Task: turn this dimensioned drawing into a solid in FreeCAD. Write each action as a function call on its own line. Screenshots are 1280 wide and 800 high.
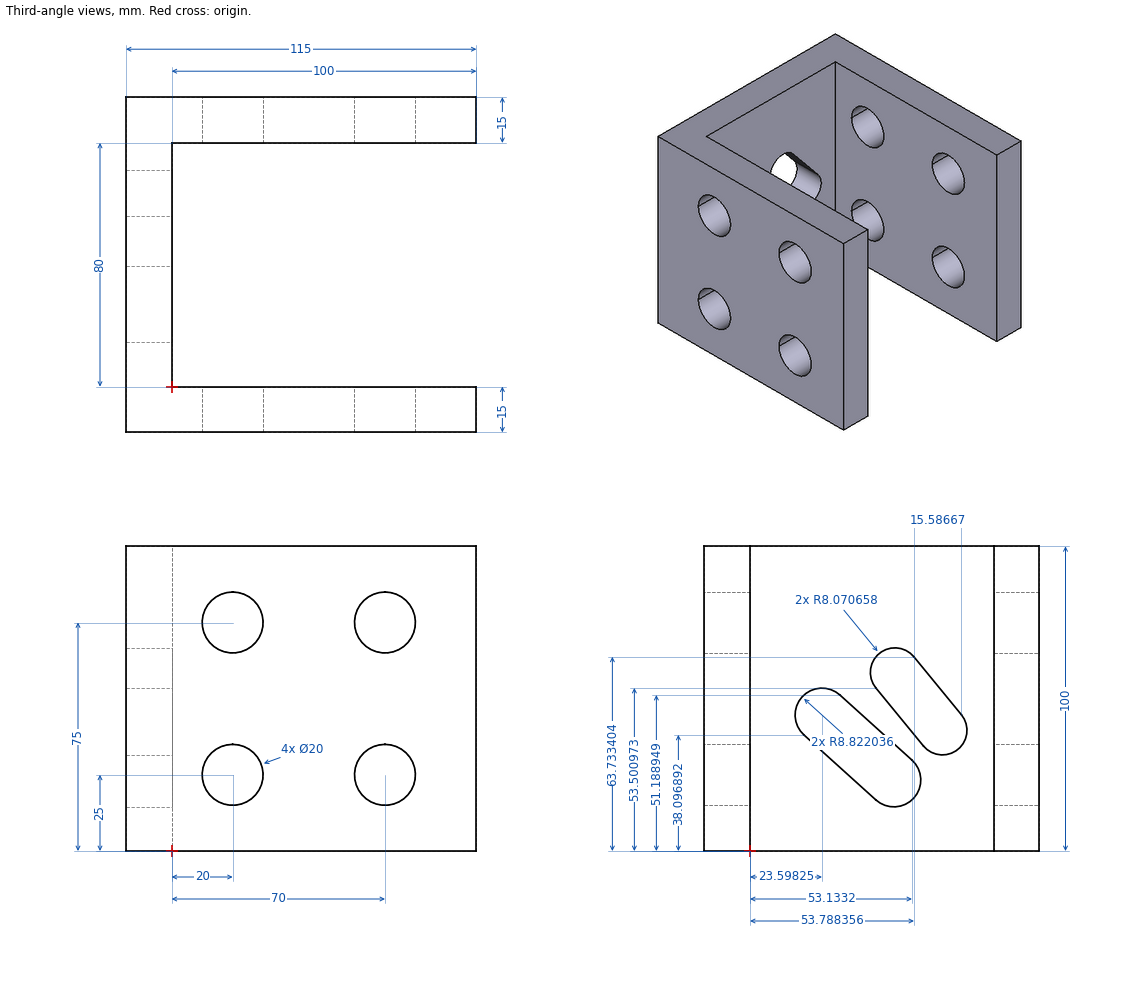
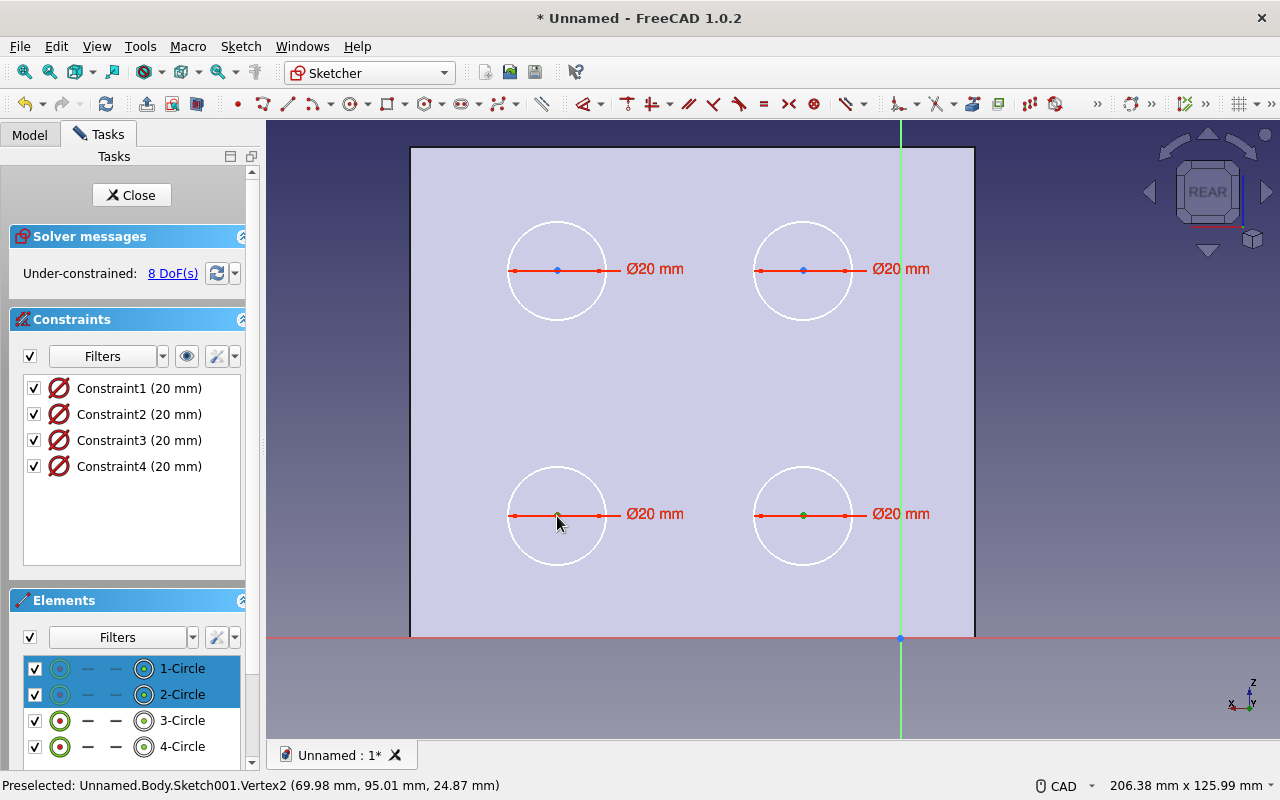
key(h)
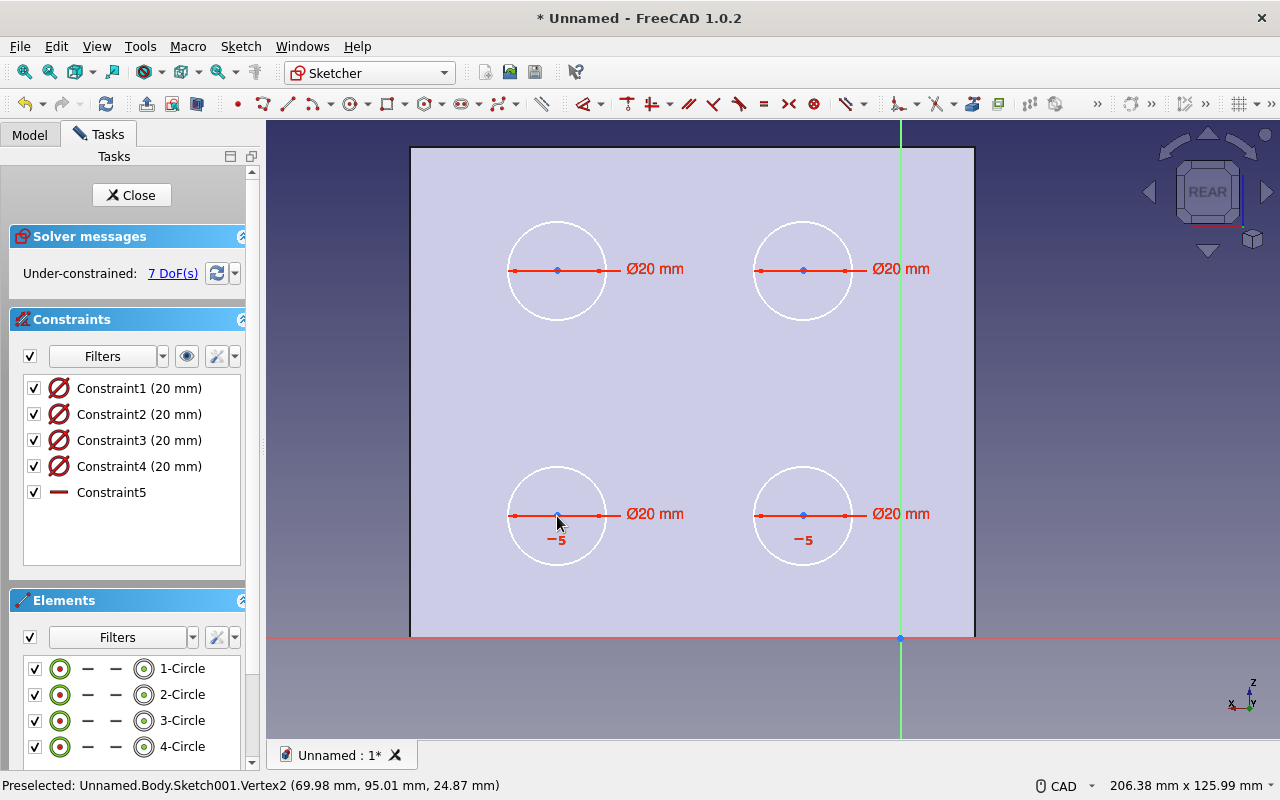
click(803, 516)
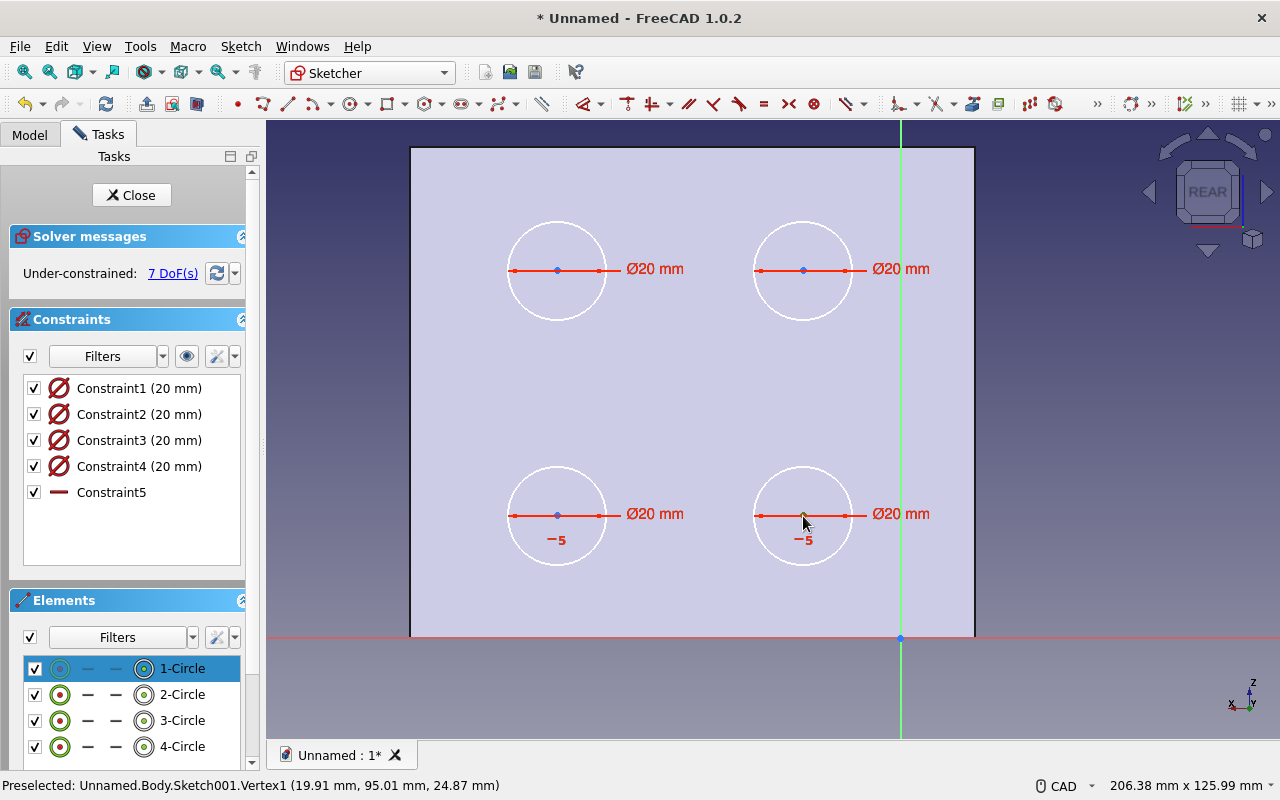
click(803, 271)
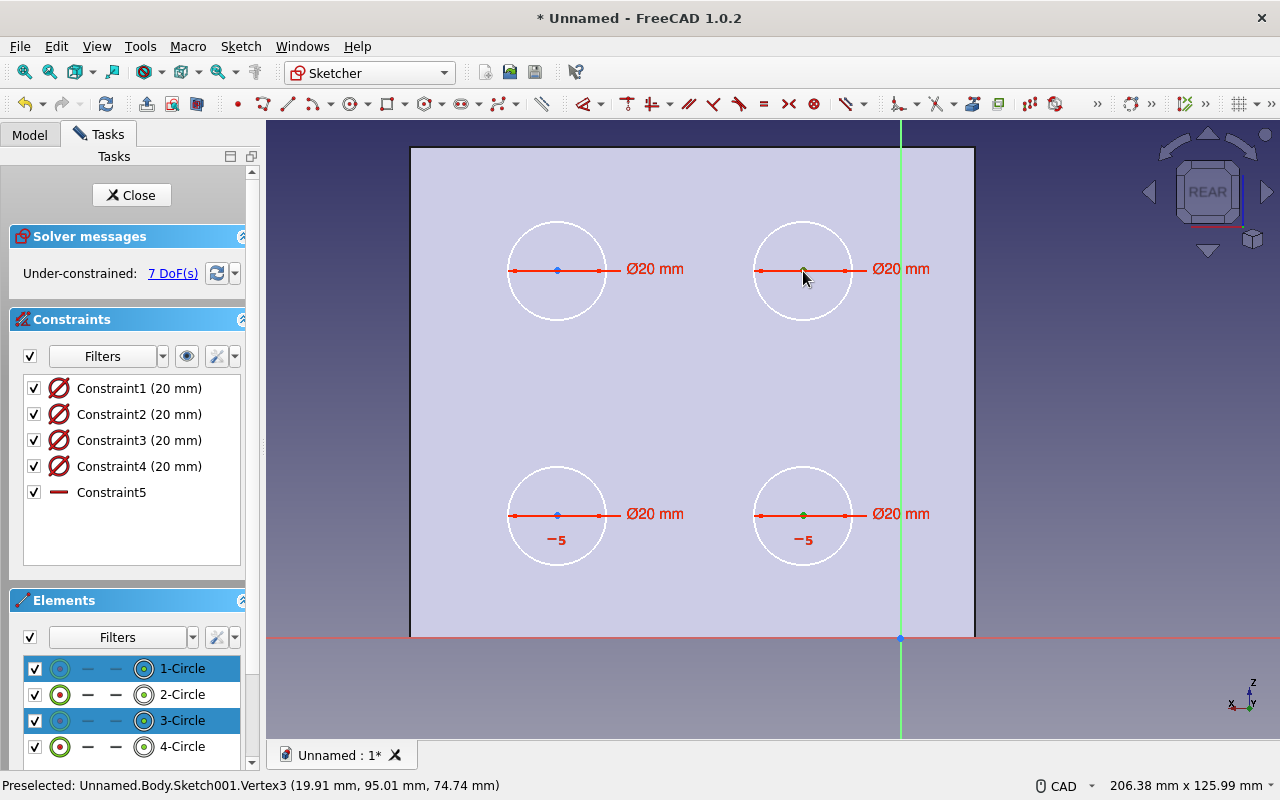
key(v)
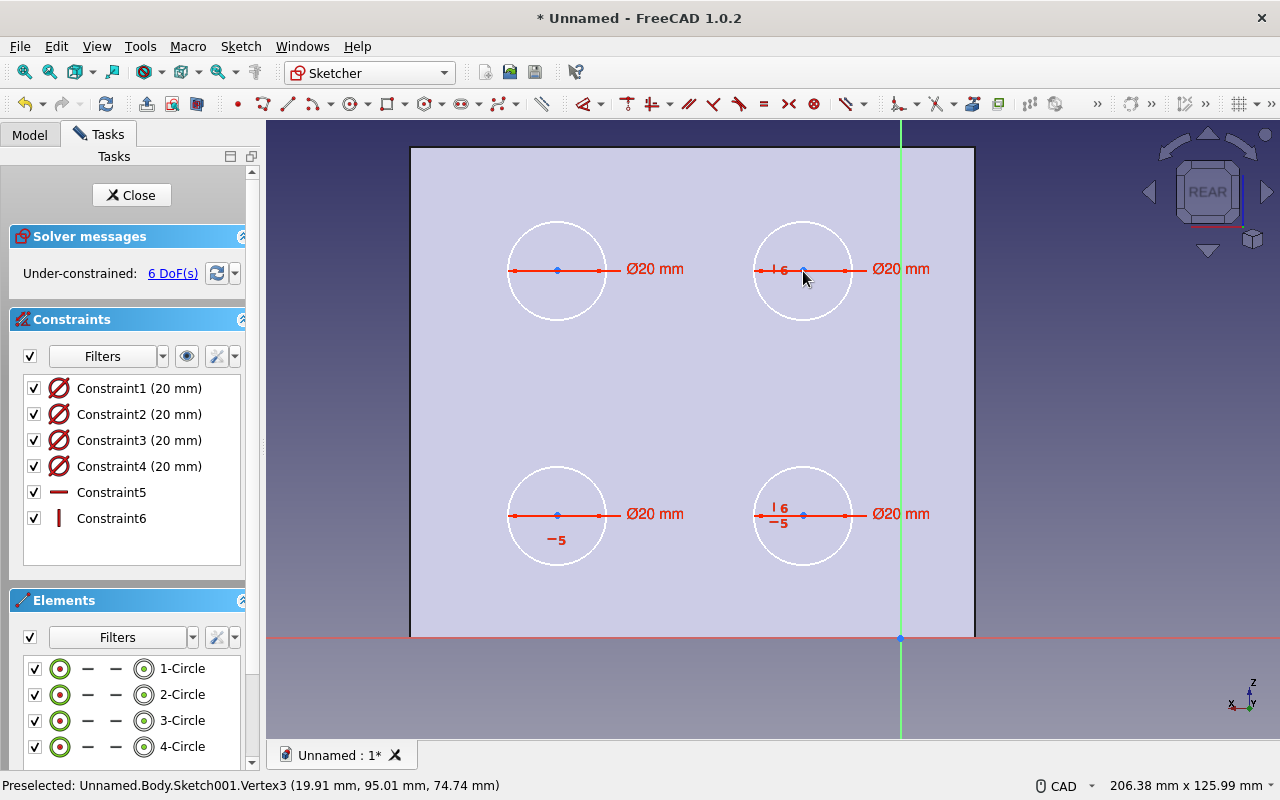
click(557, 516)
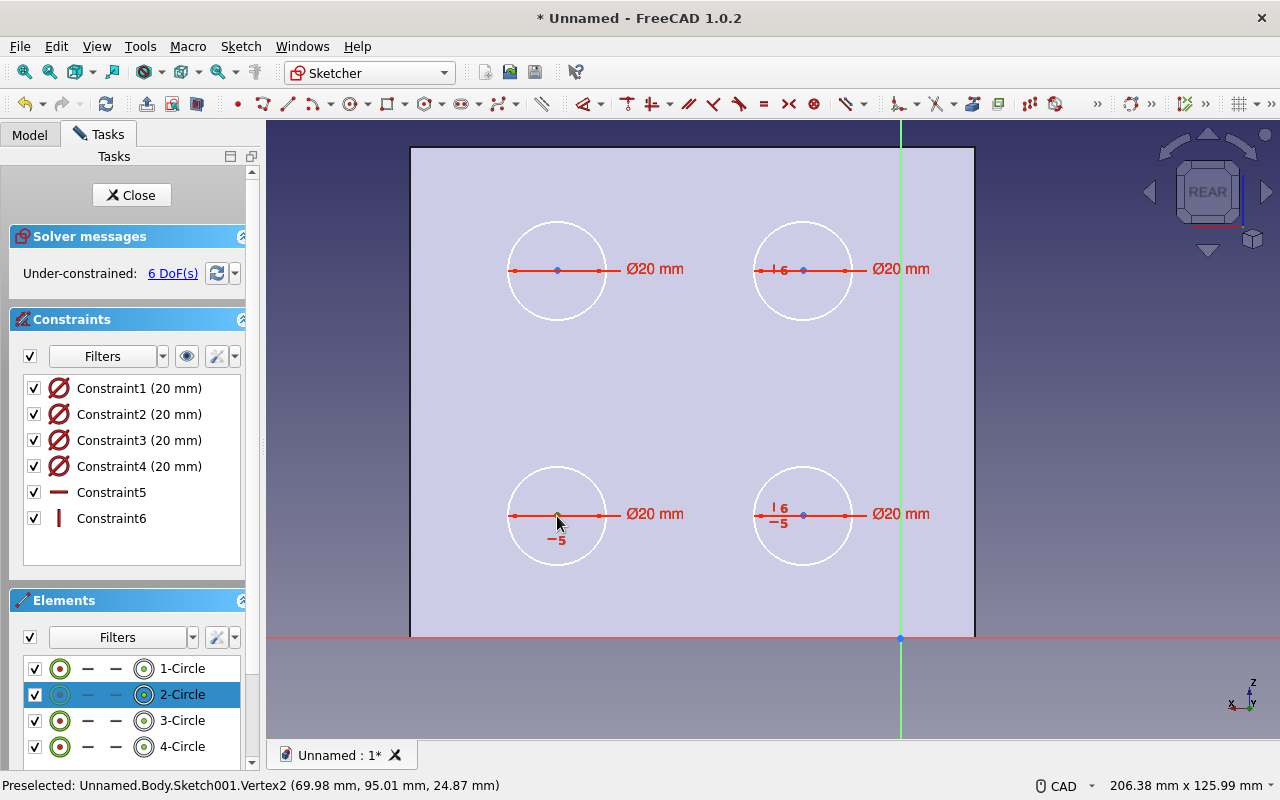
click(557, 271)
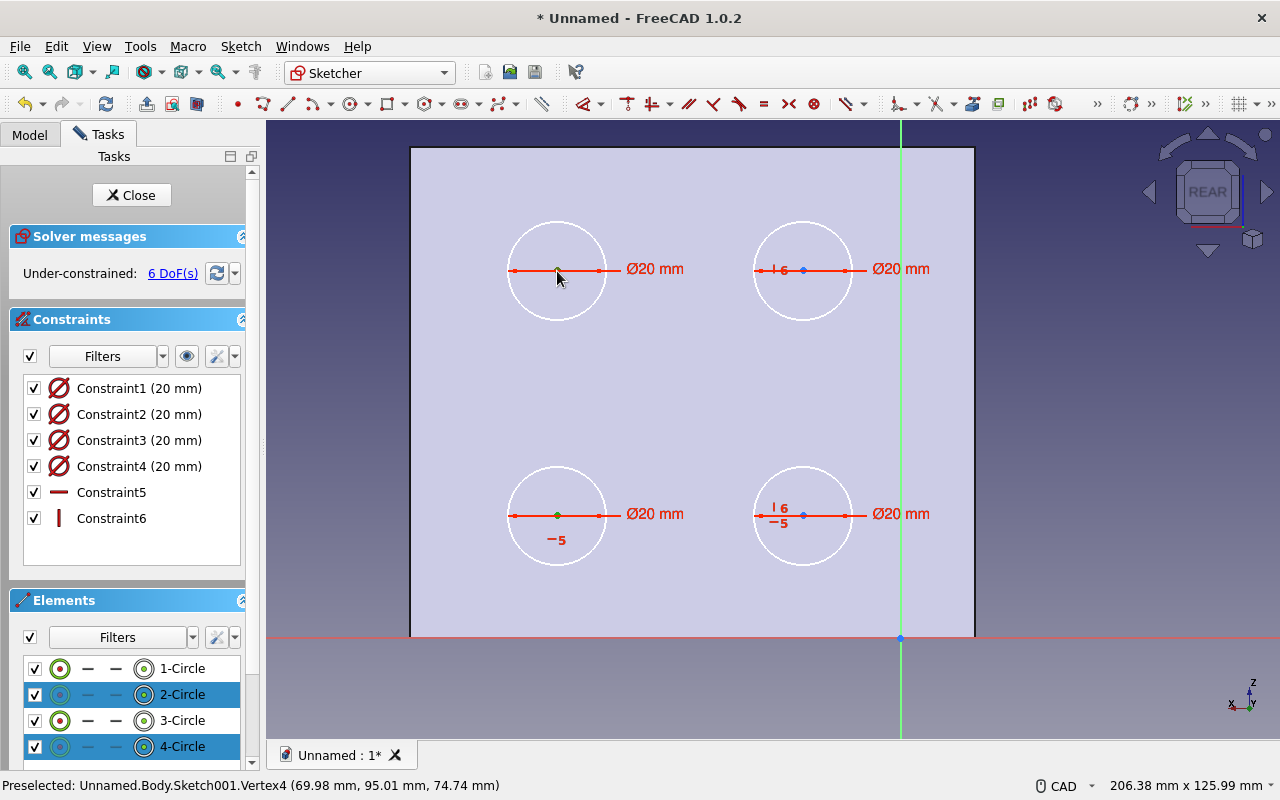
click(670, 104)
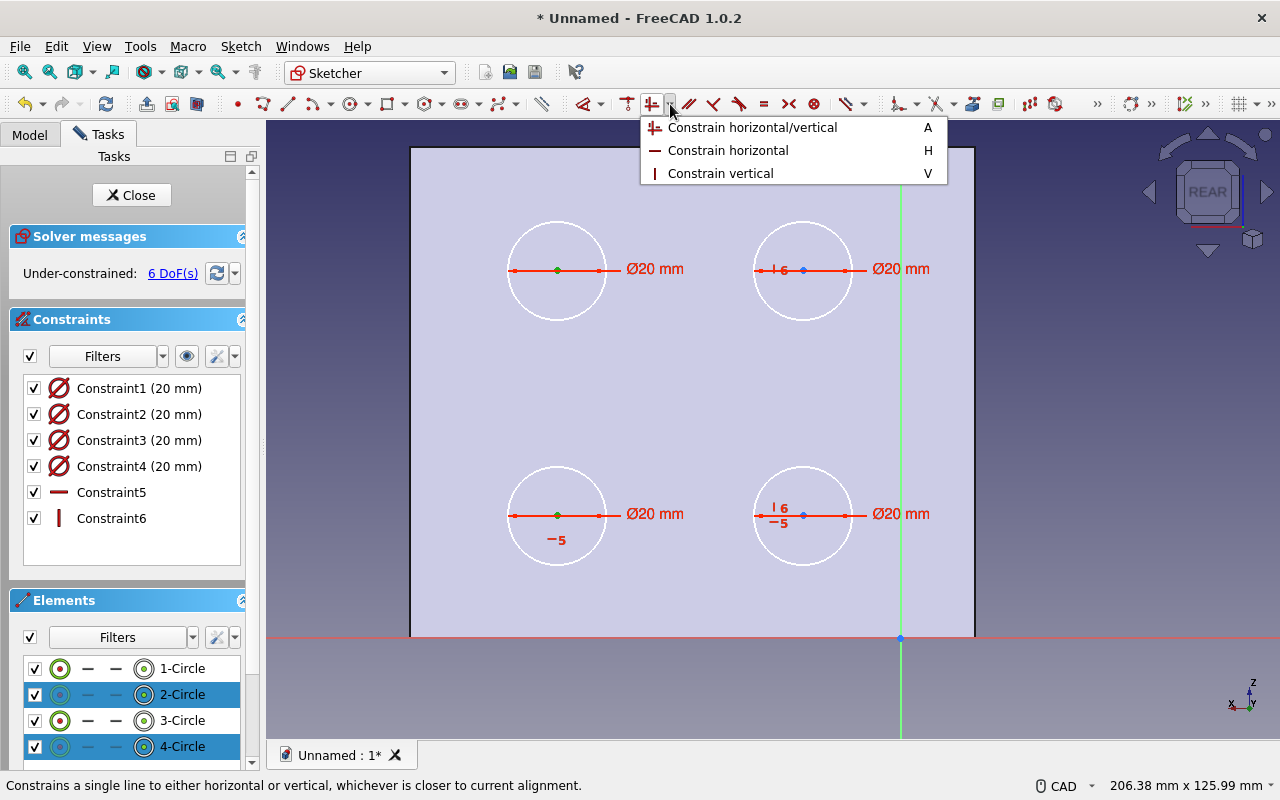
click(794, 174)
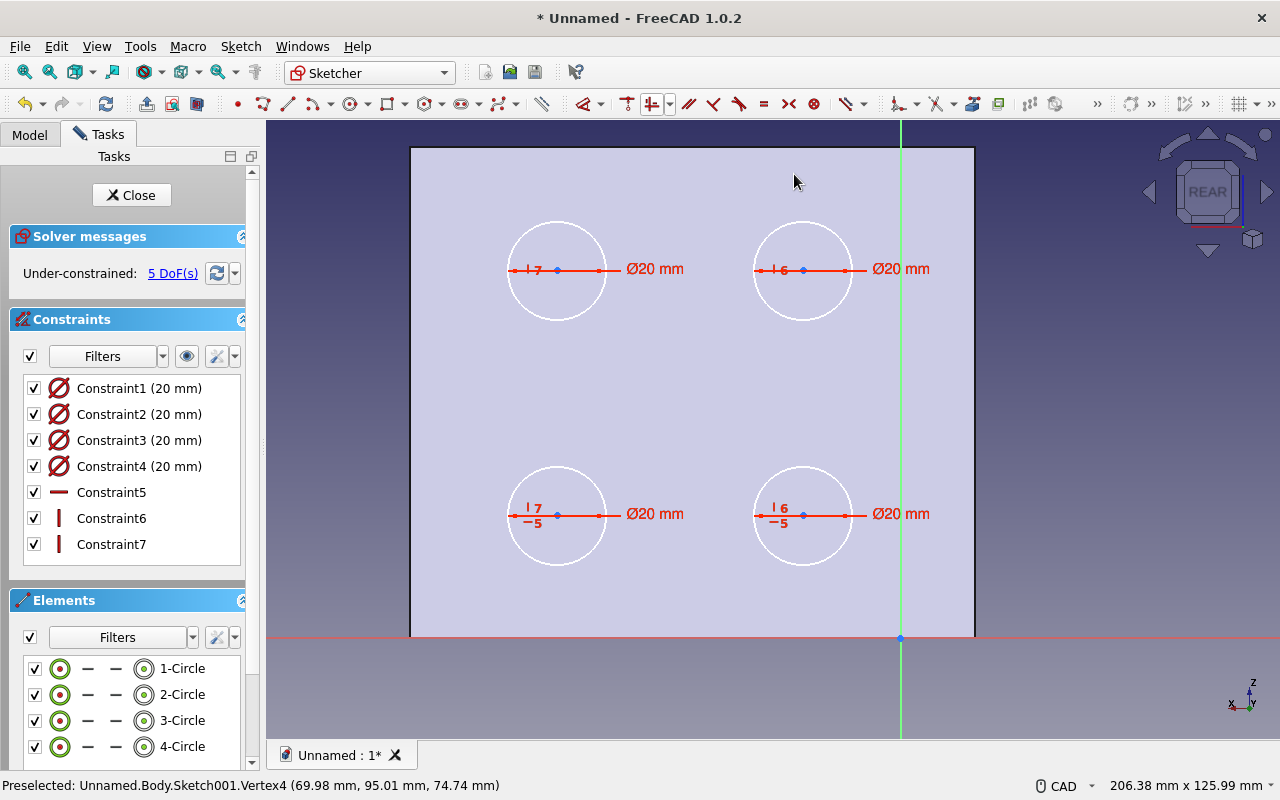
click(803, 271)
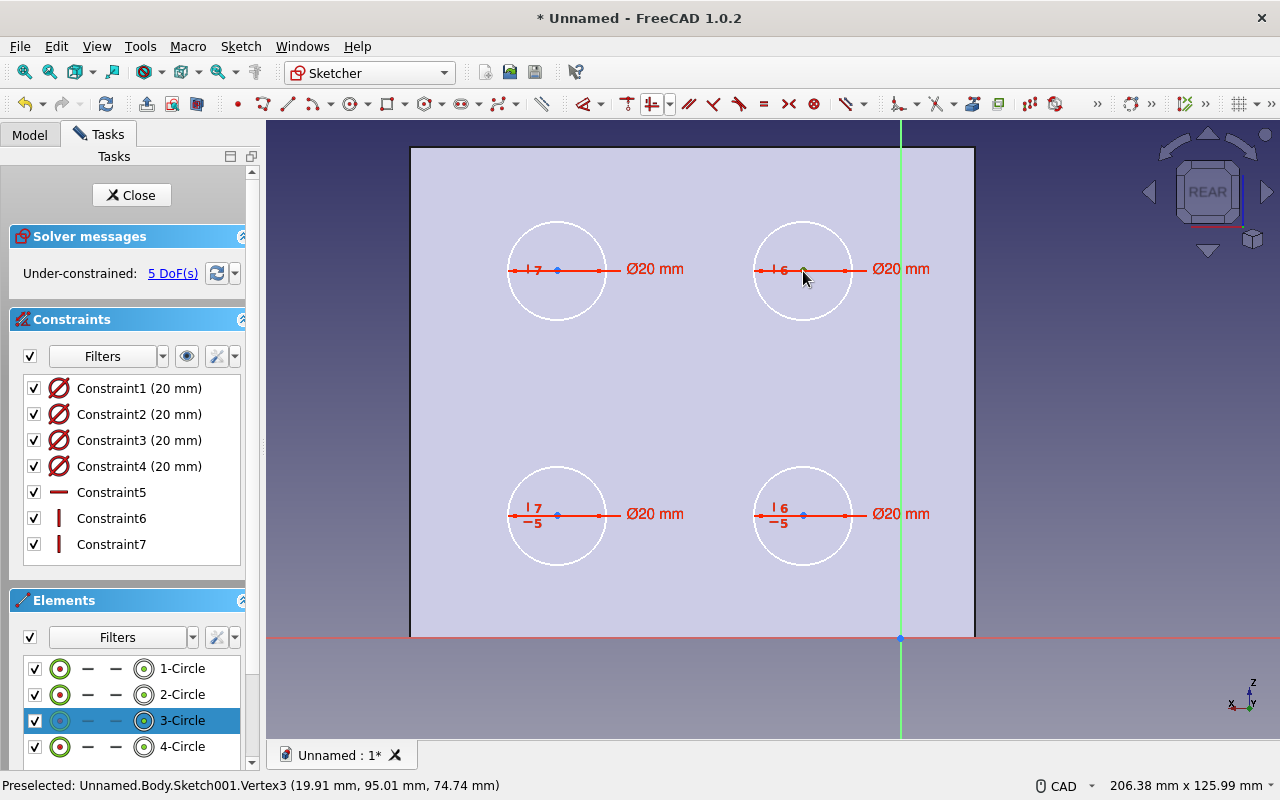
click(557, 271)